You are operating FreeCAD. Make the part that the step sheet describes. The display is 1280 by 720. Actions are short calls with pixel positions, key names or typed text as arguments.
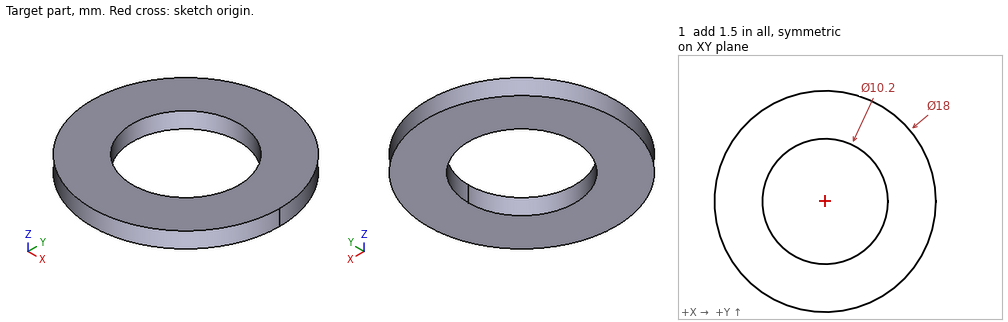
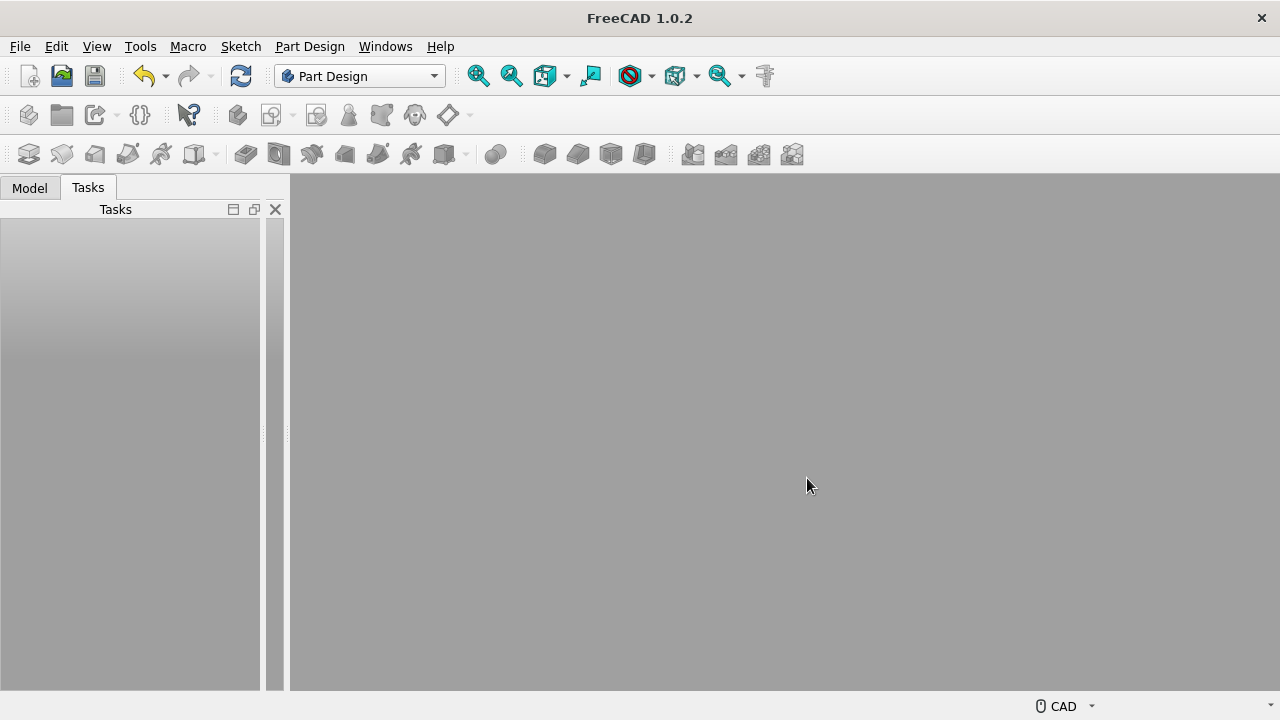
click(29, 76)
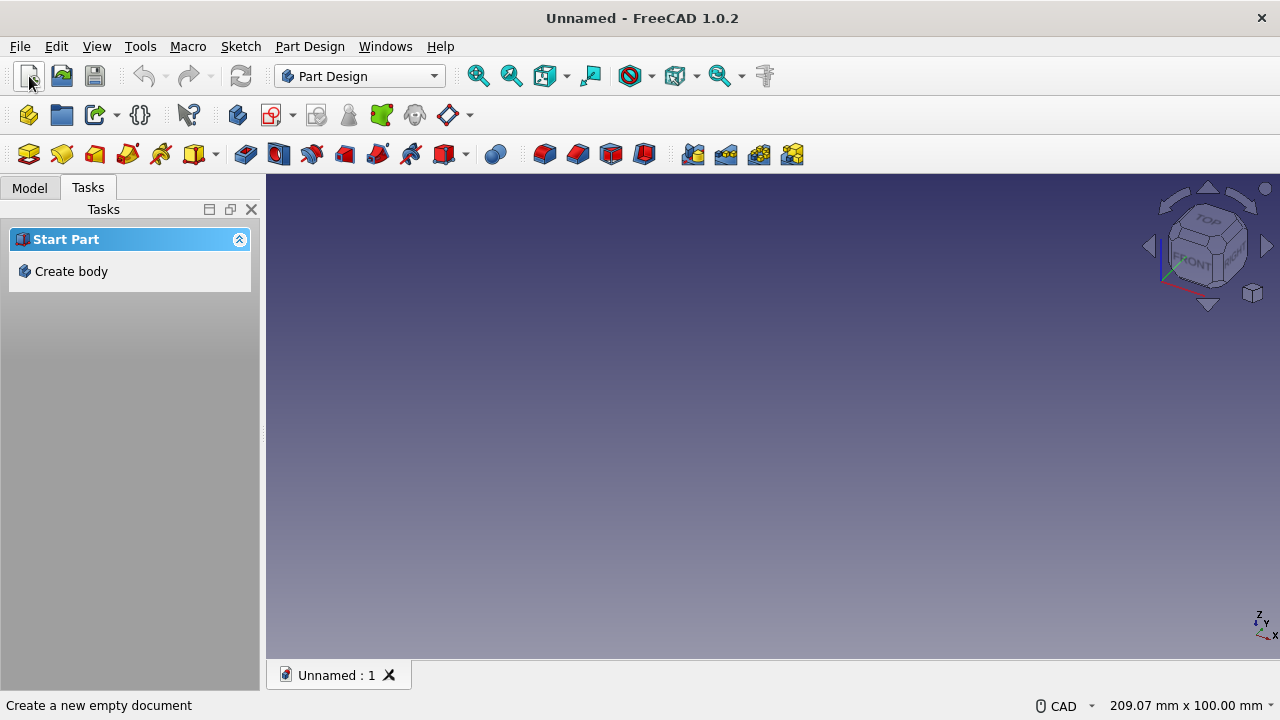
click(270, 116)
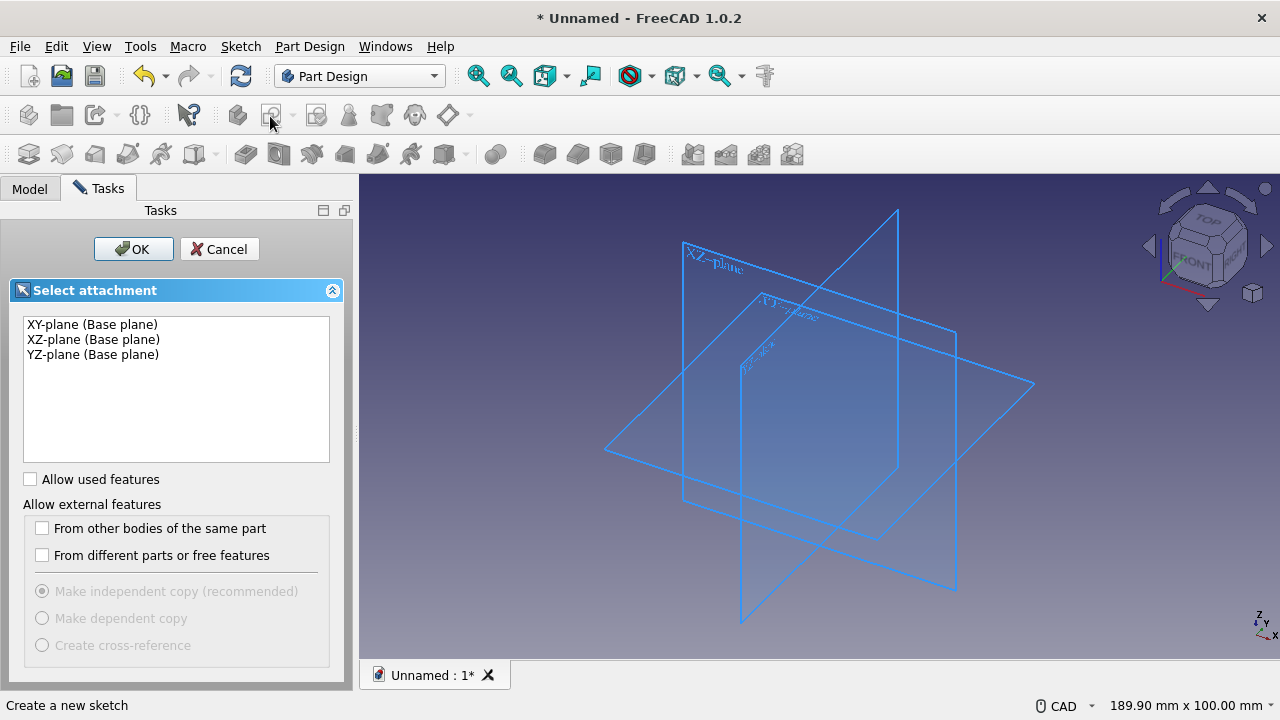
click(84, 324)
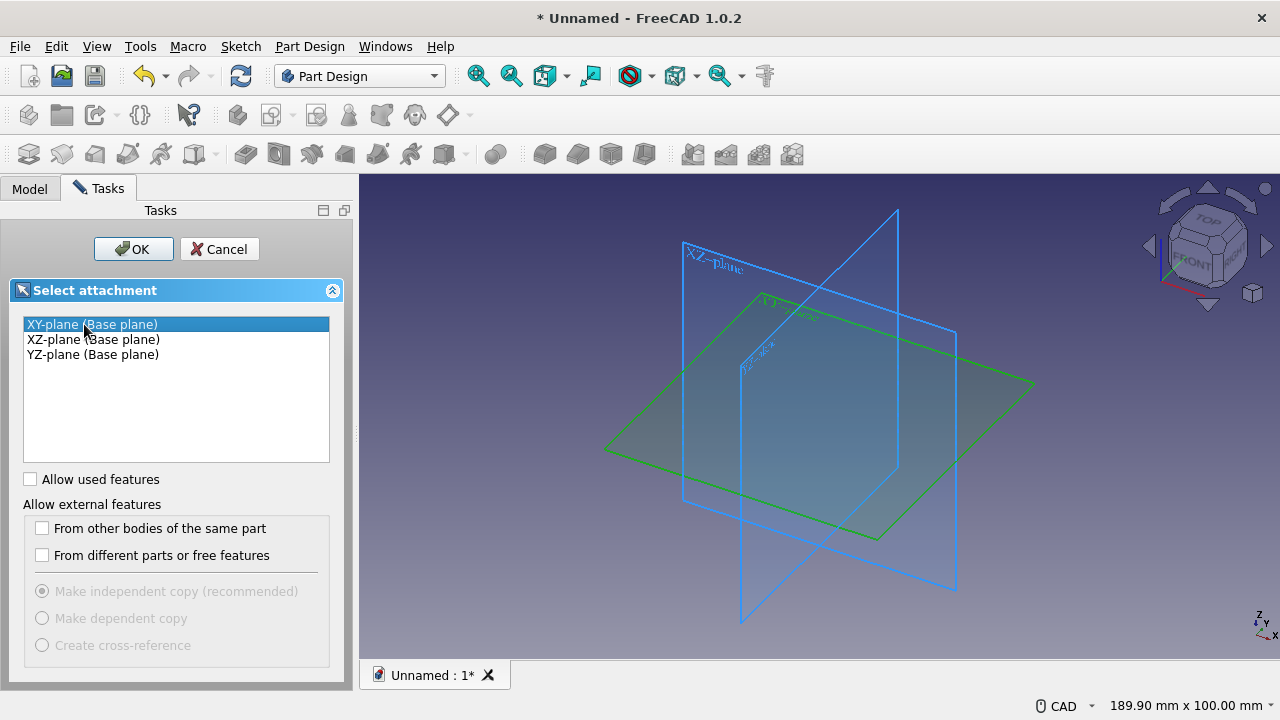
click(134, 249)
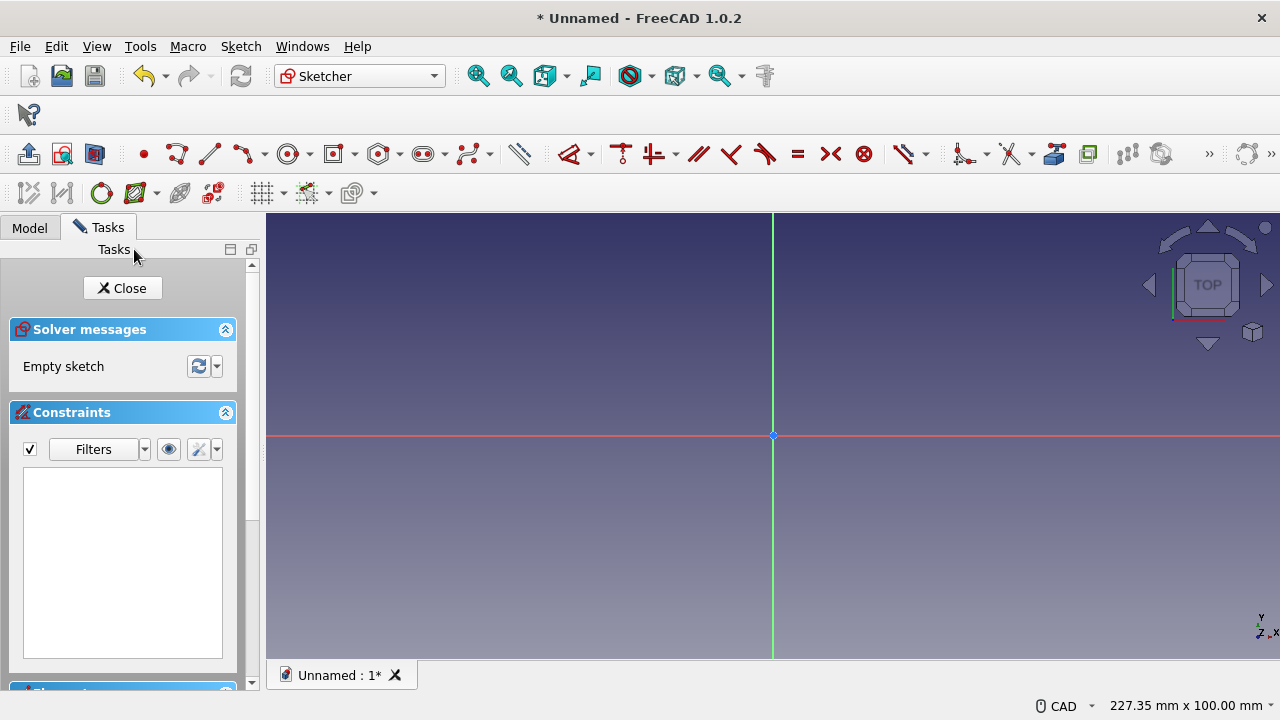
scroll(803, 436, up, 6)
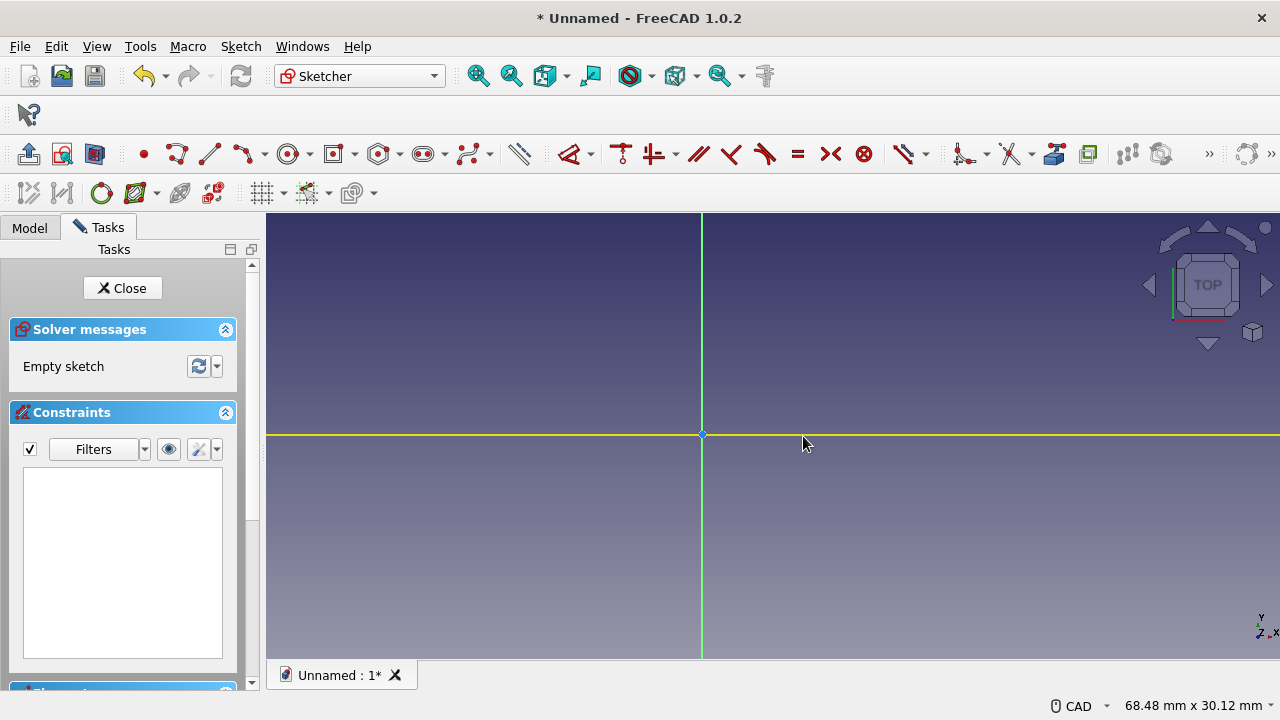
click(288, 154)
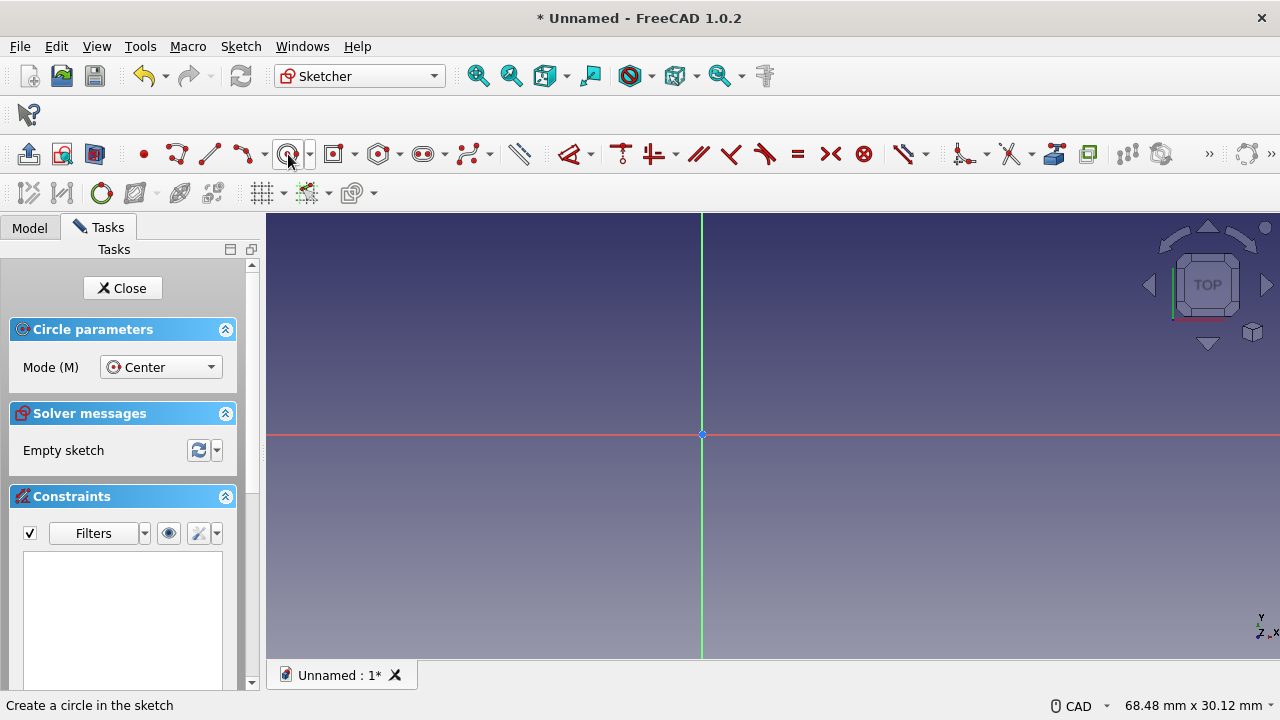
click(702, 435)
click(796, 341)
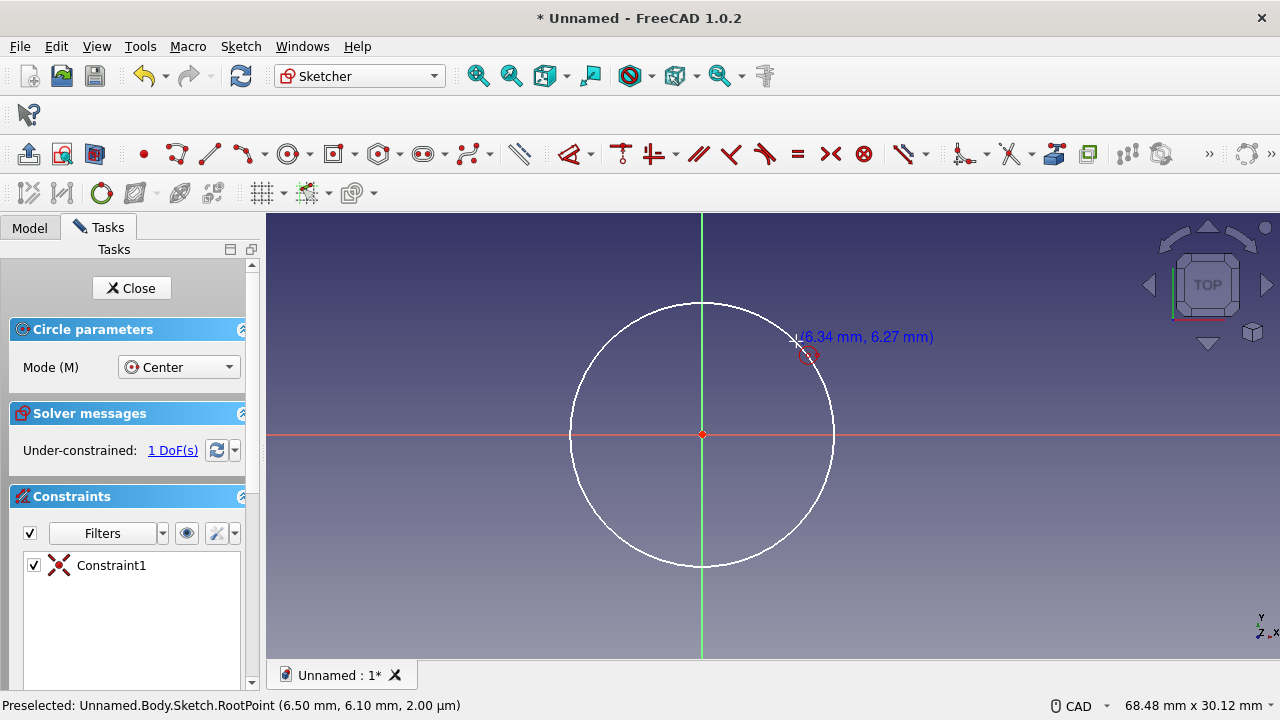
click(702, 435)
click(756, 381)
key(Escape)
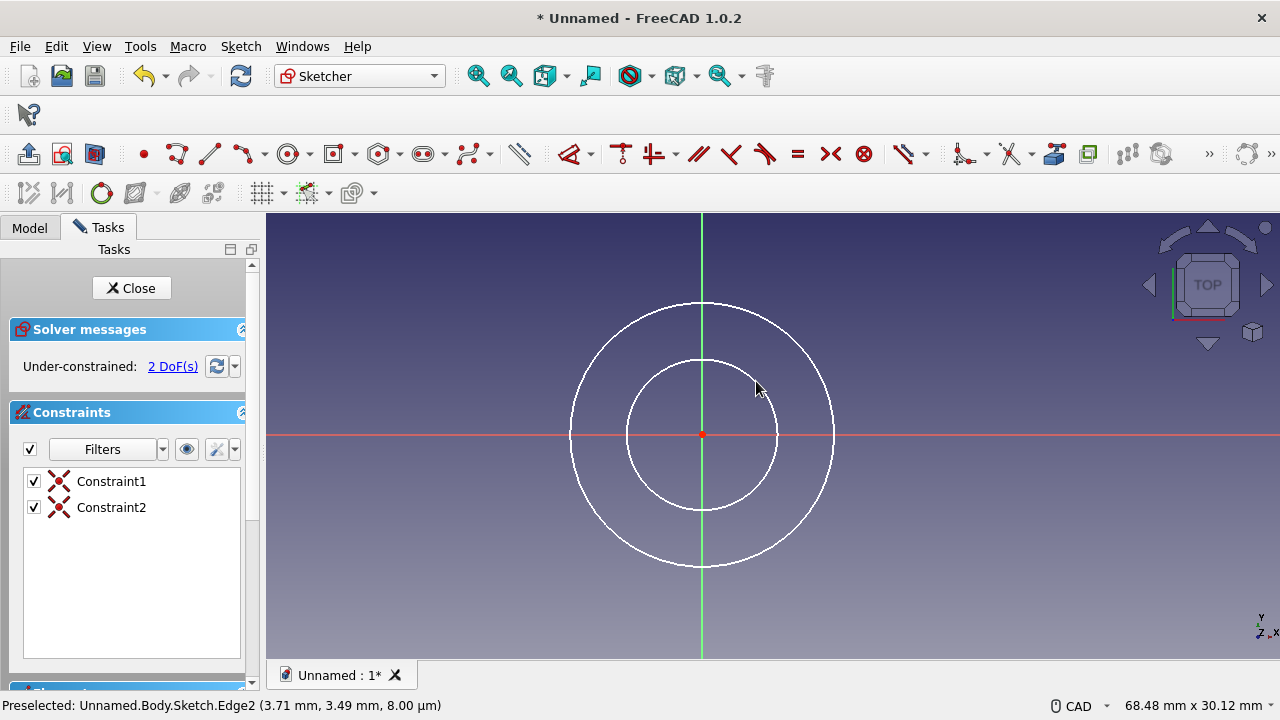
click(568, 154)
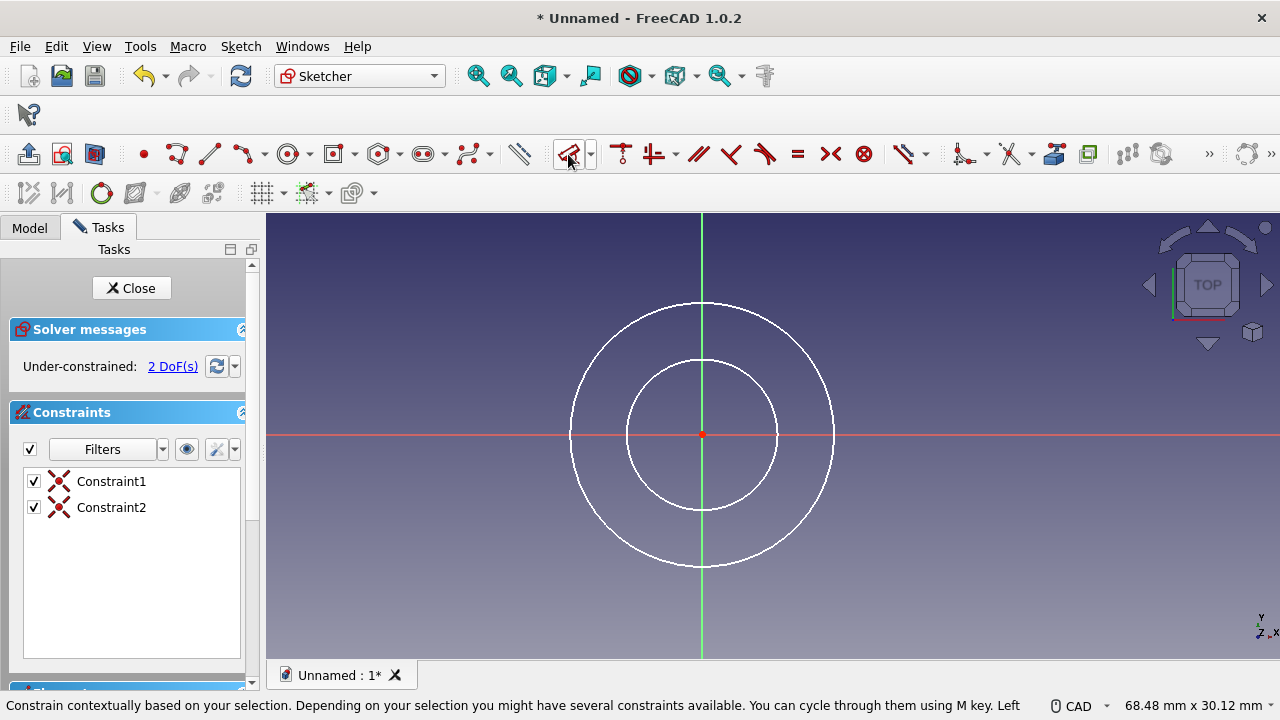
click(795, 341)
click(818, 318)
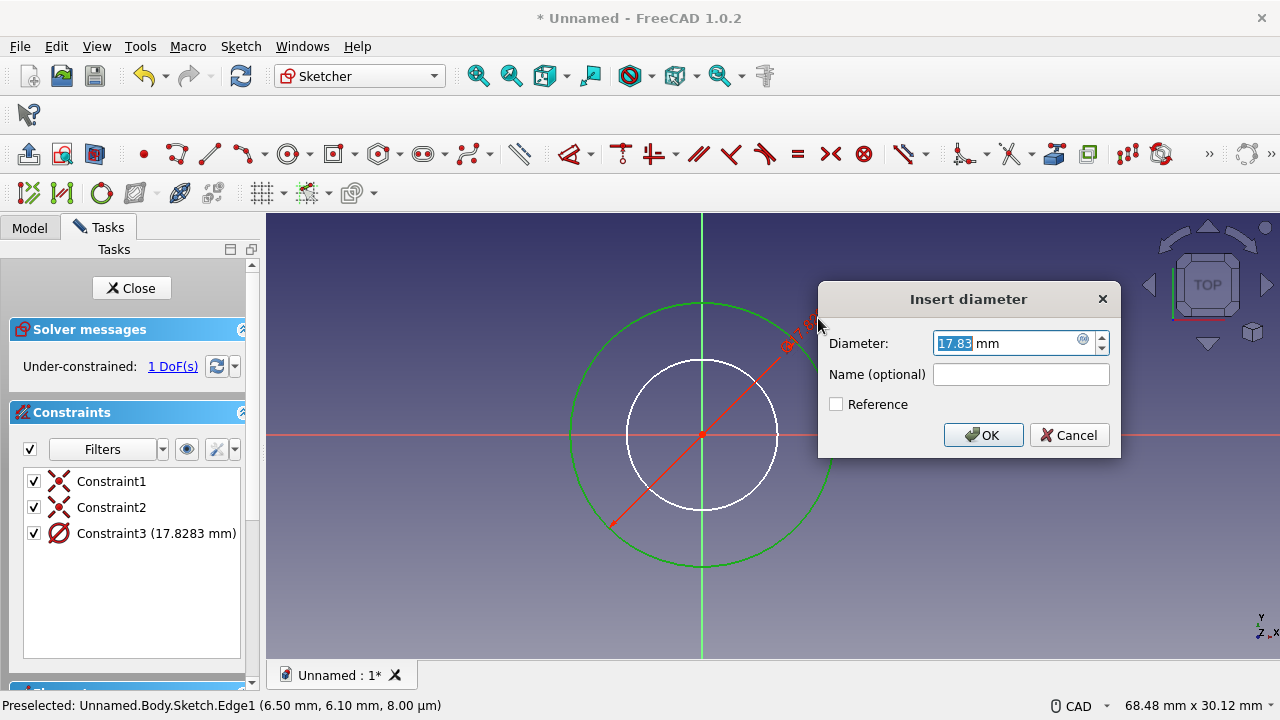
text(18)
key(Return)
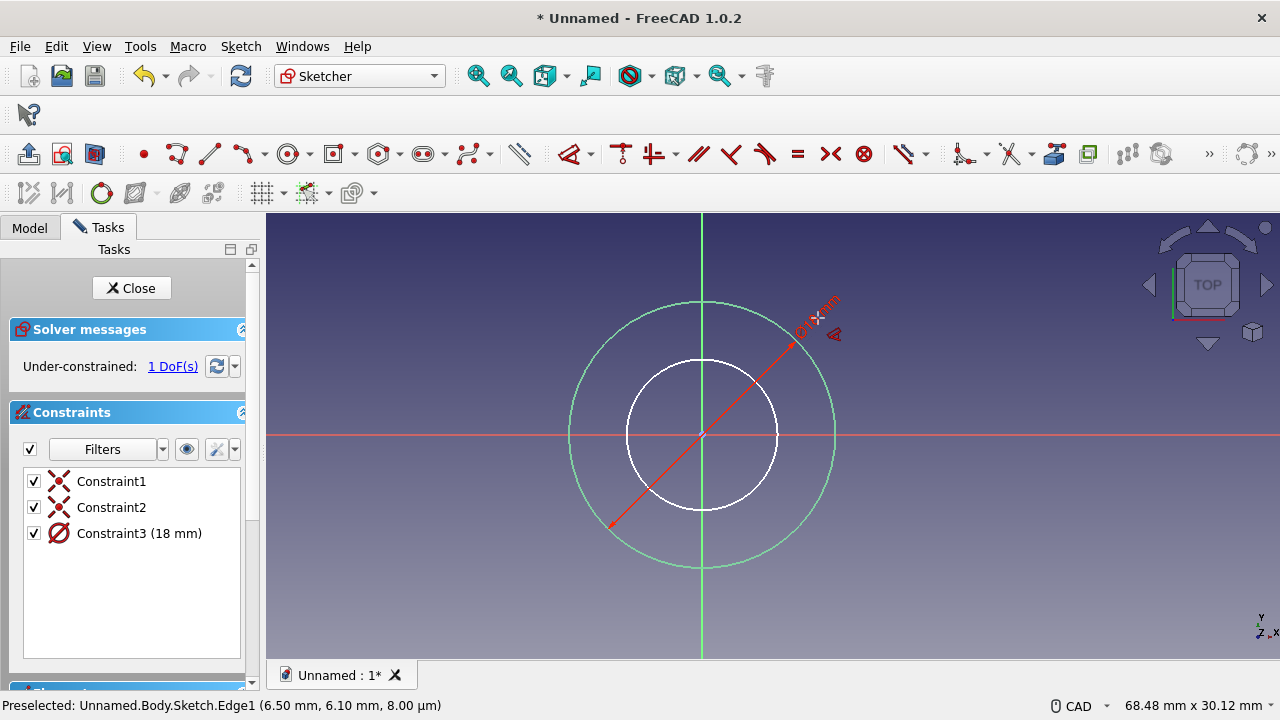
click(755, 381)
click(777, 358)